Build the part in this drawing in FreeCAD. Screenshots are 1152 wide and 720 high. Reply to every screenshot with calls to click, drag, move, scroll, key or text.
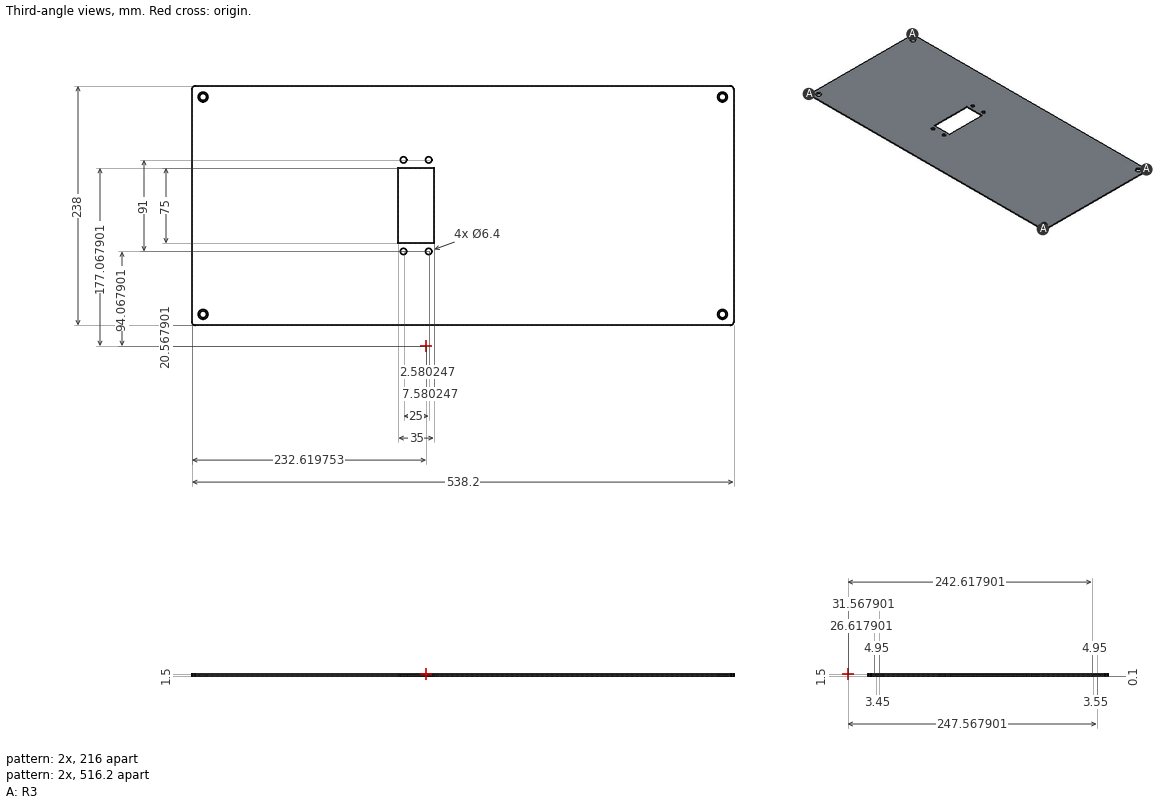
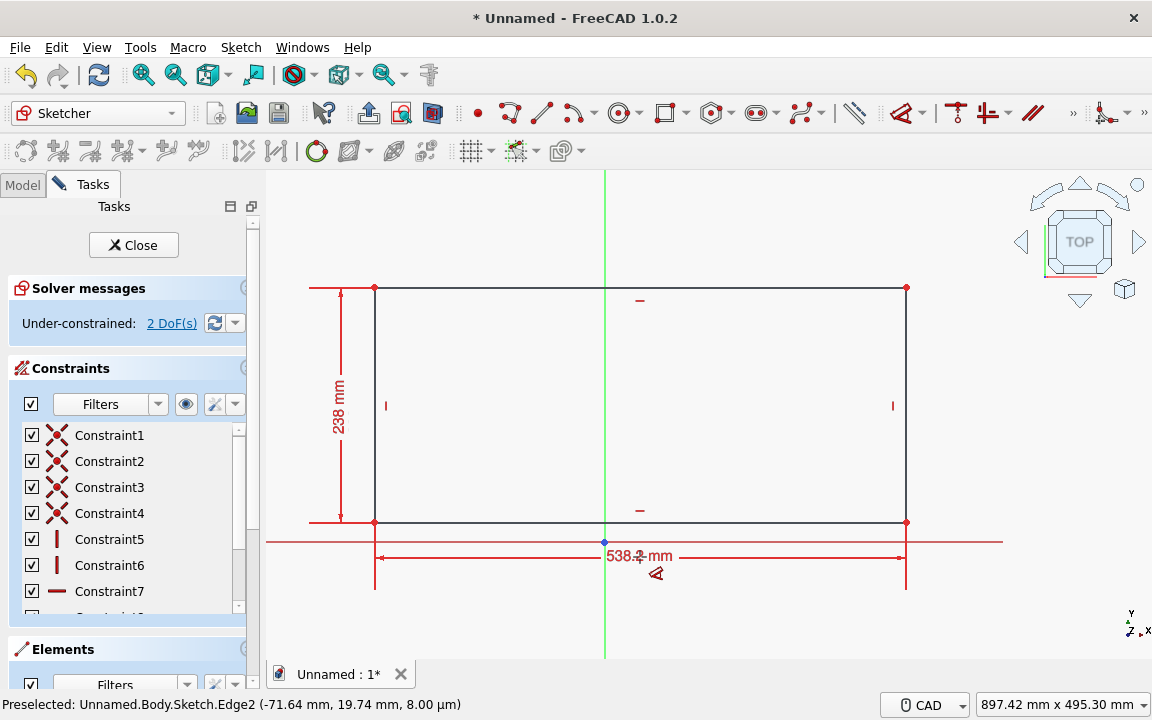
scroll(375, 523, up, 4)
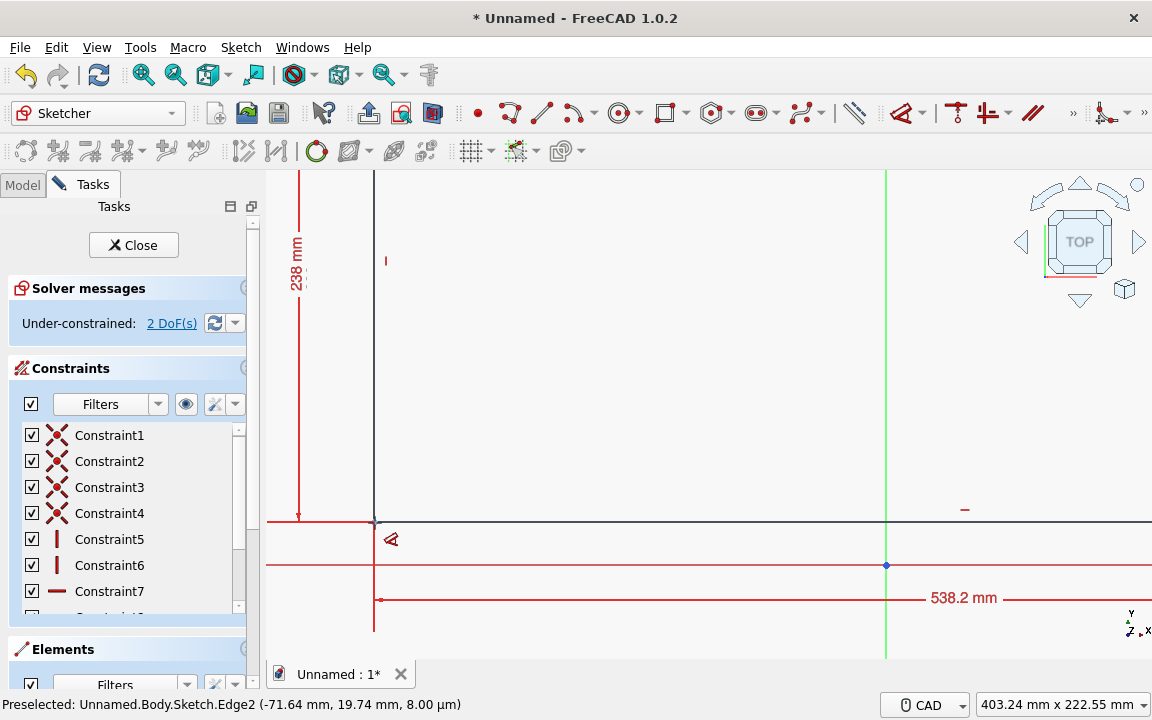
click(374, 522)
click(340, 544)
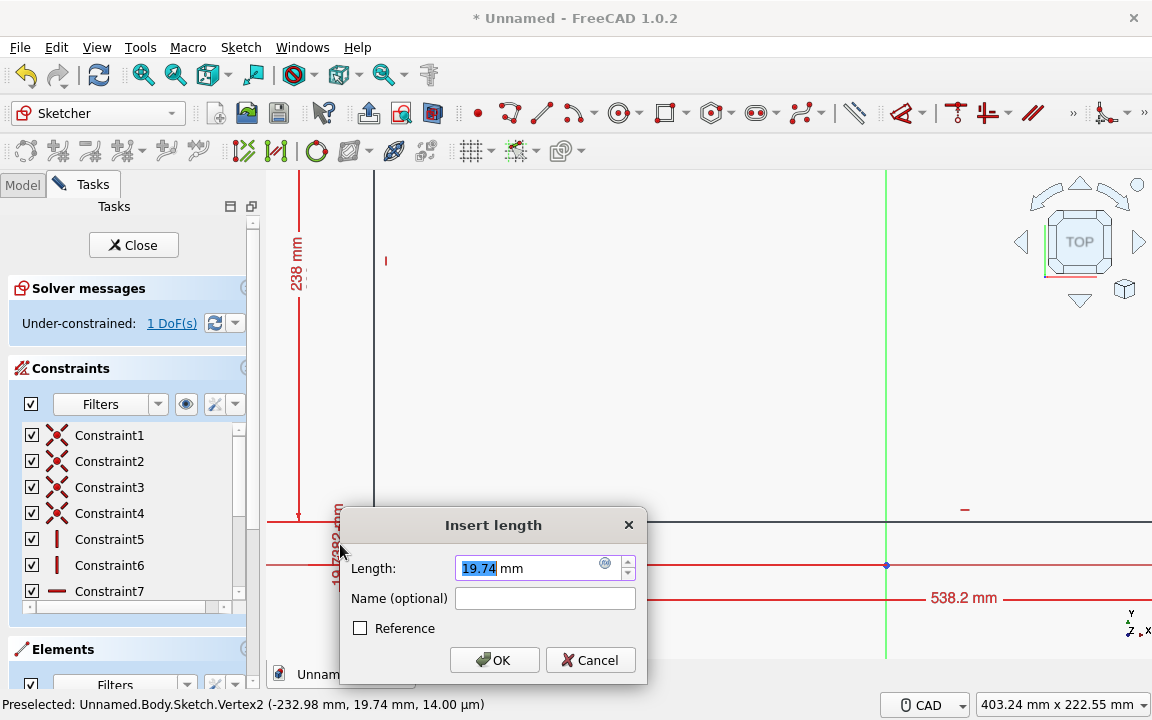
text(20.567901)
key(Return)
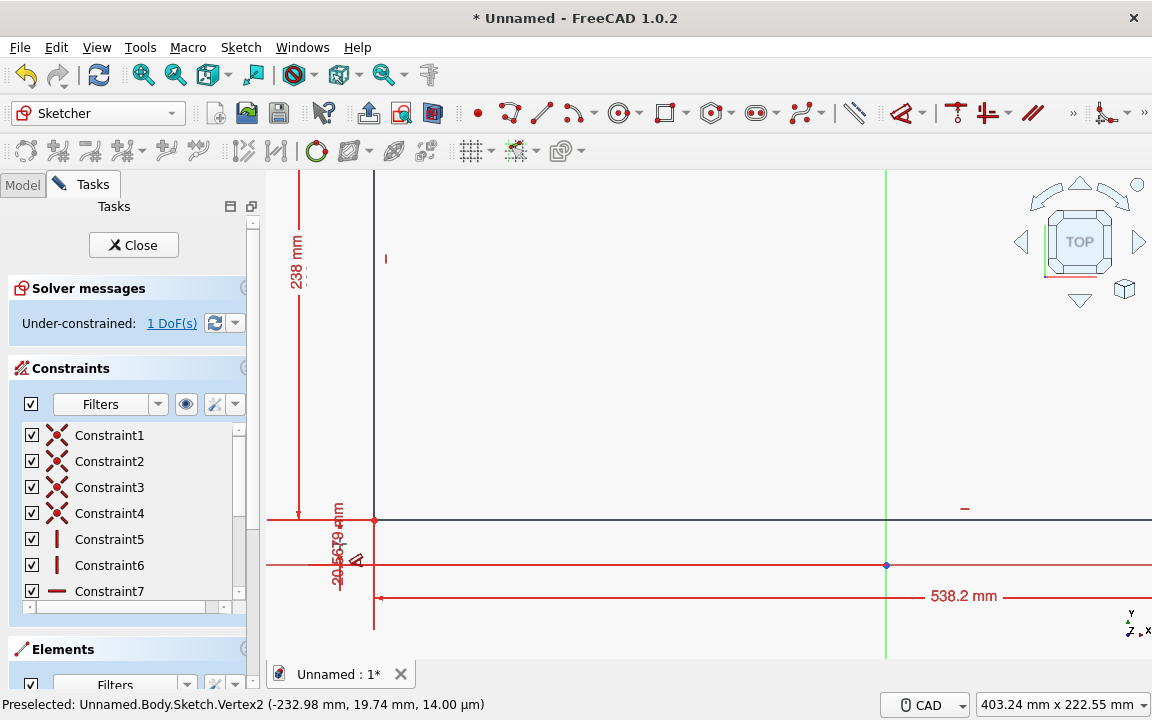
scroll(375, 523, down, 4)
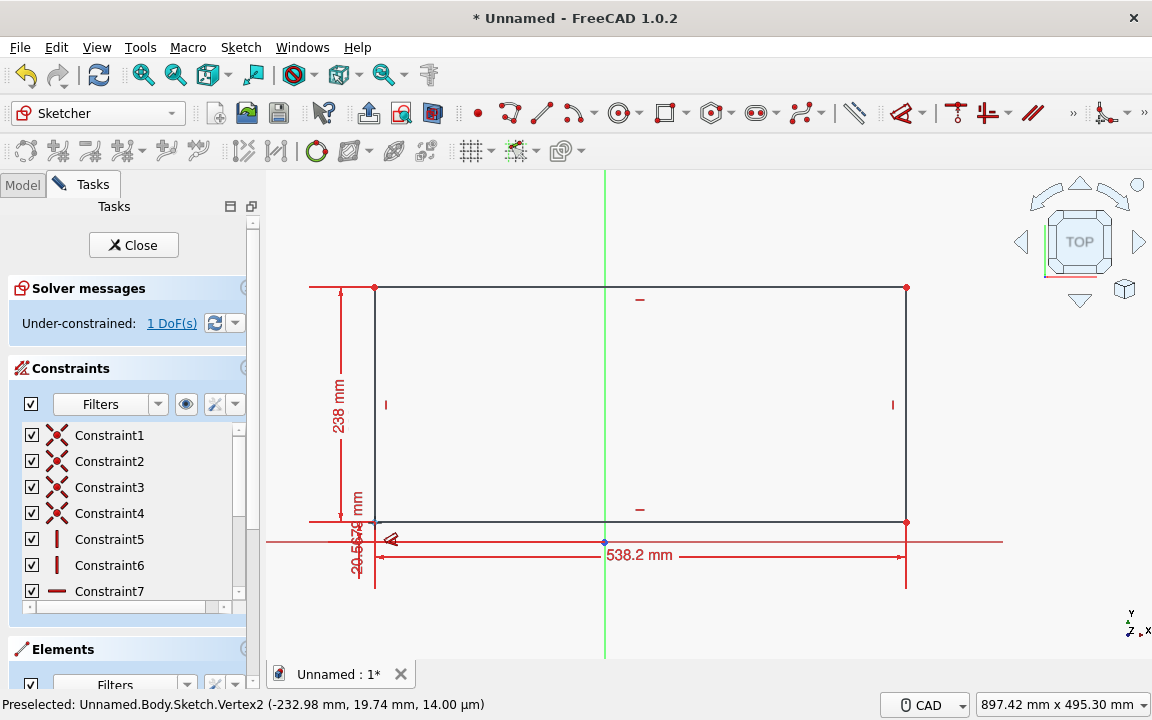
click(375, 287)
click(490, 576)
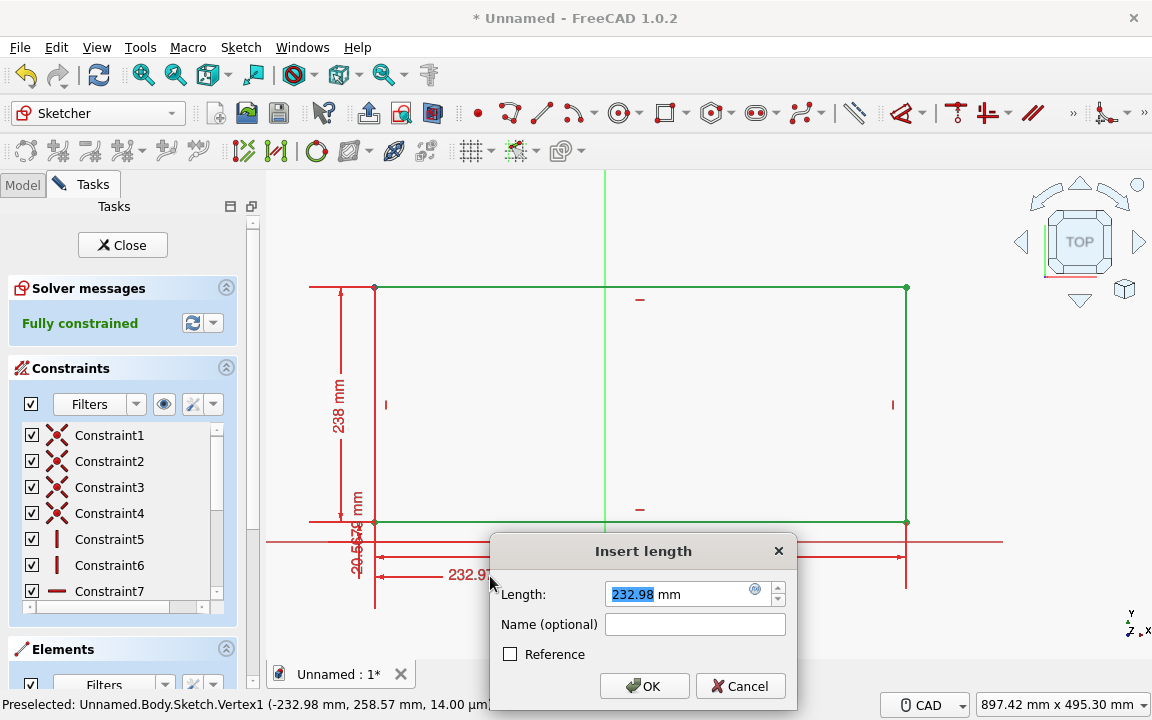
text(232.619753)
key(Return)
key(Escape)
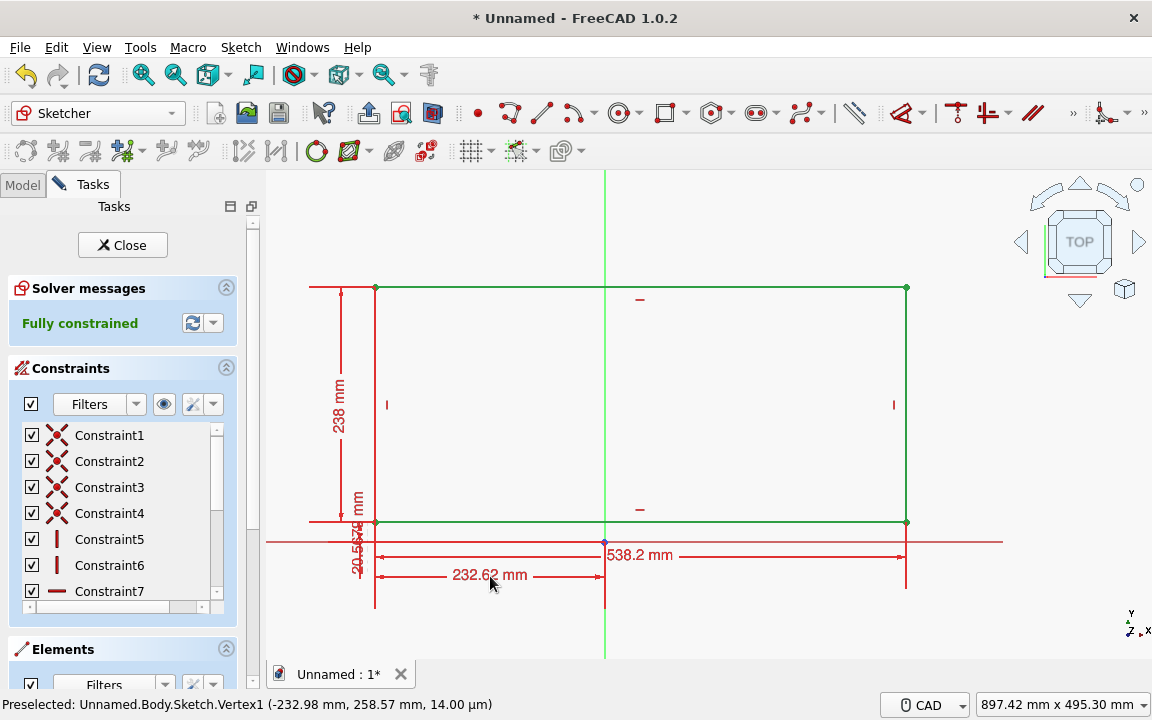
click(123, 245)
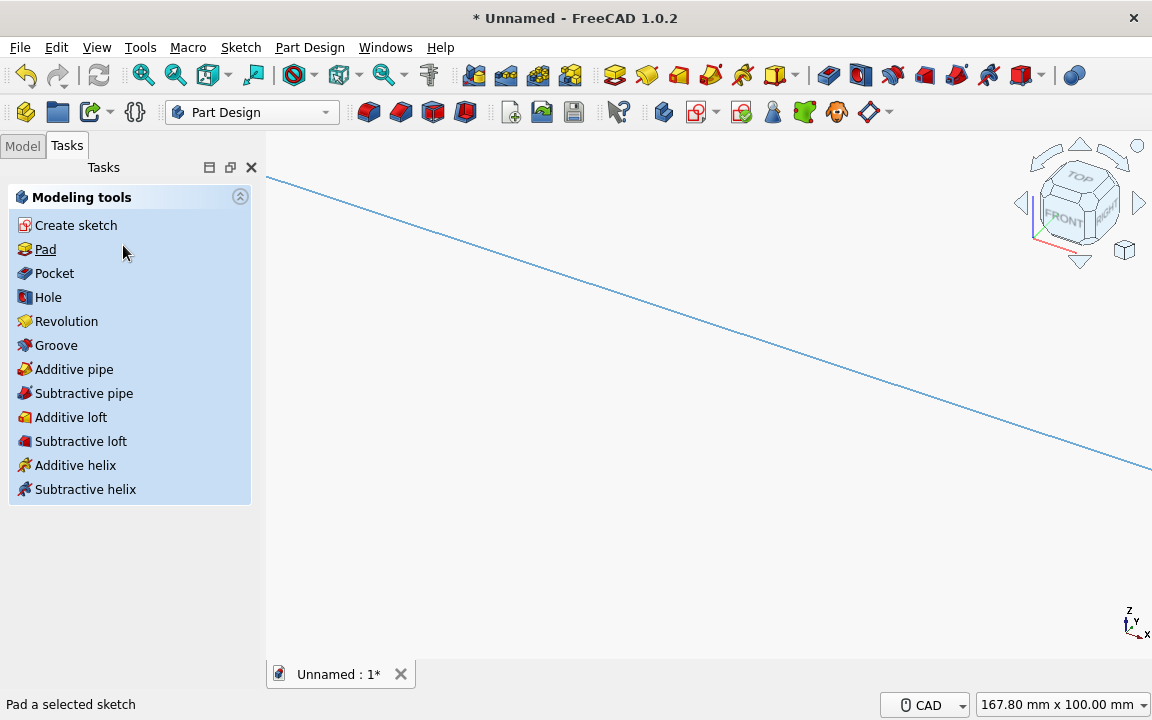
click(616, 76)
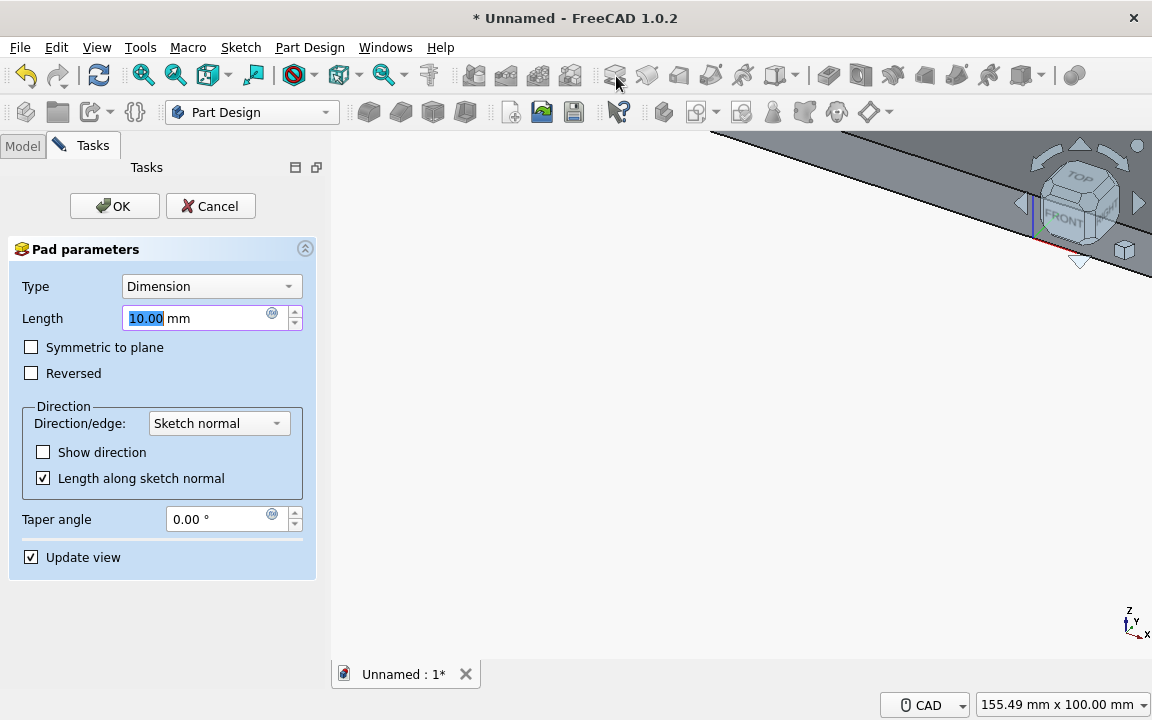
text(1.5)
key(Tab)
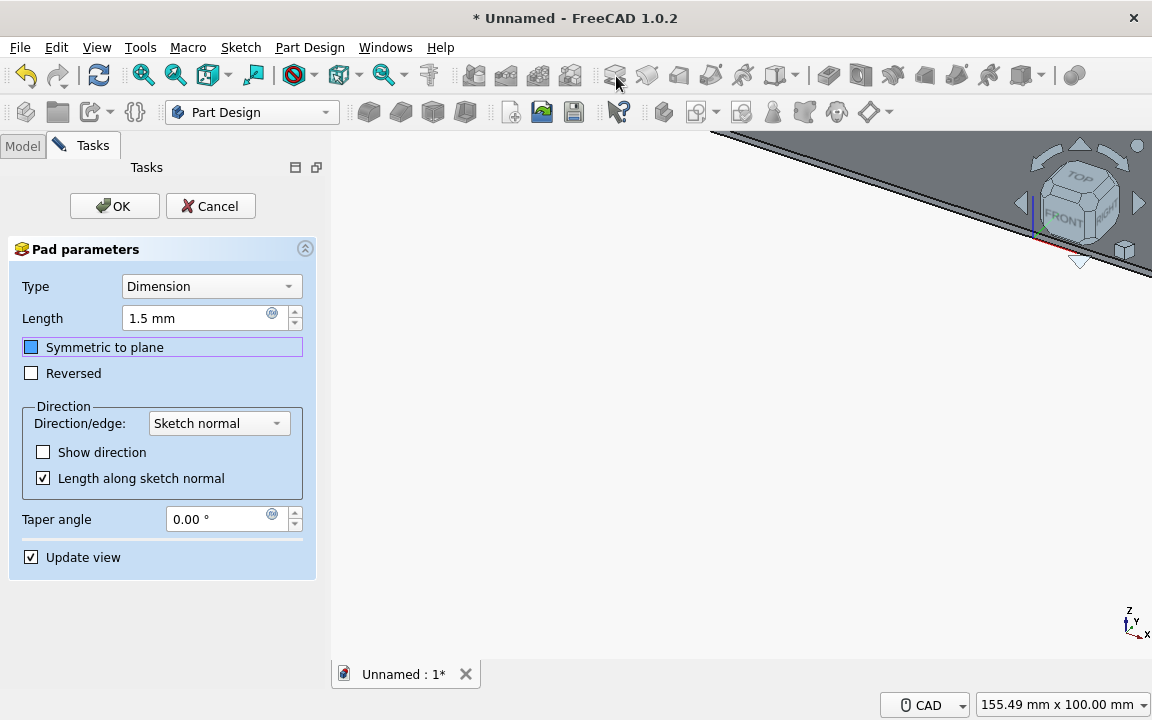
click(30, 373)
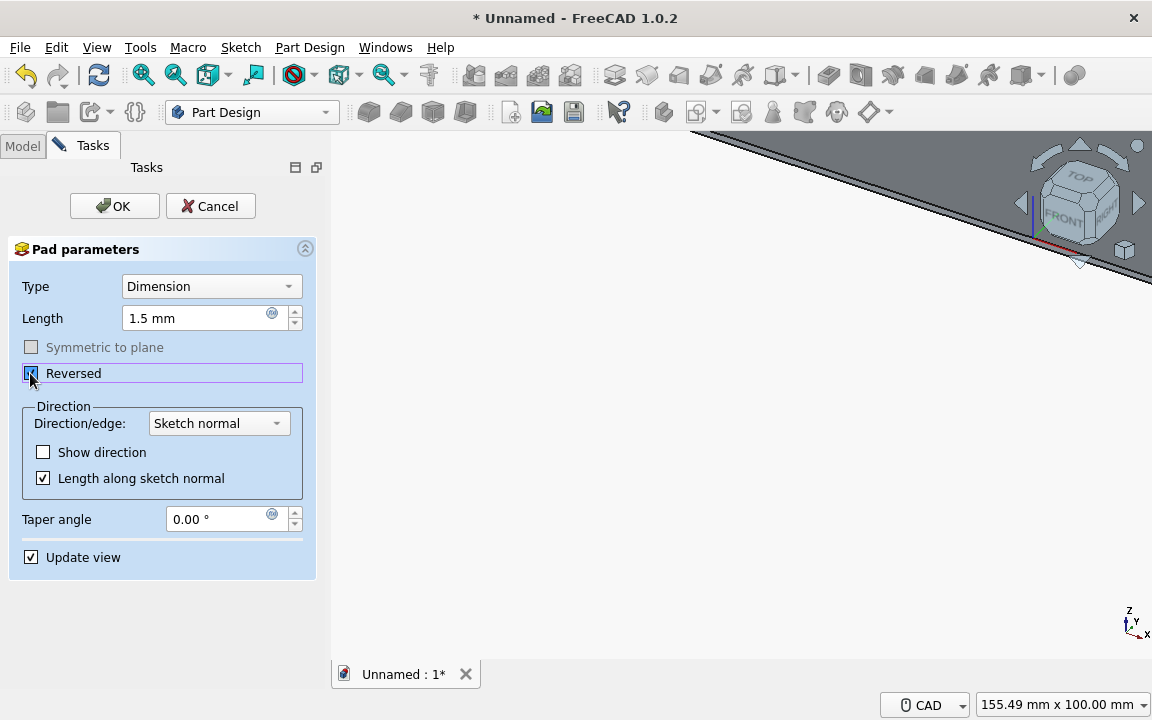
click(115, 206)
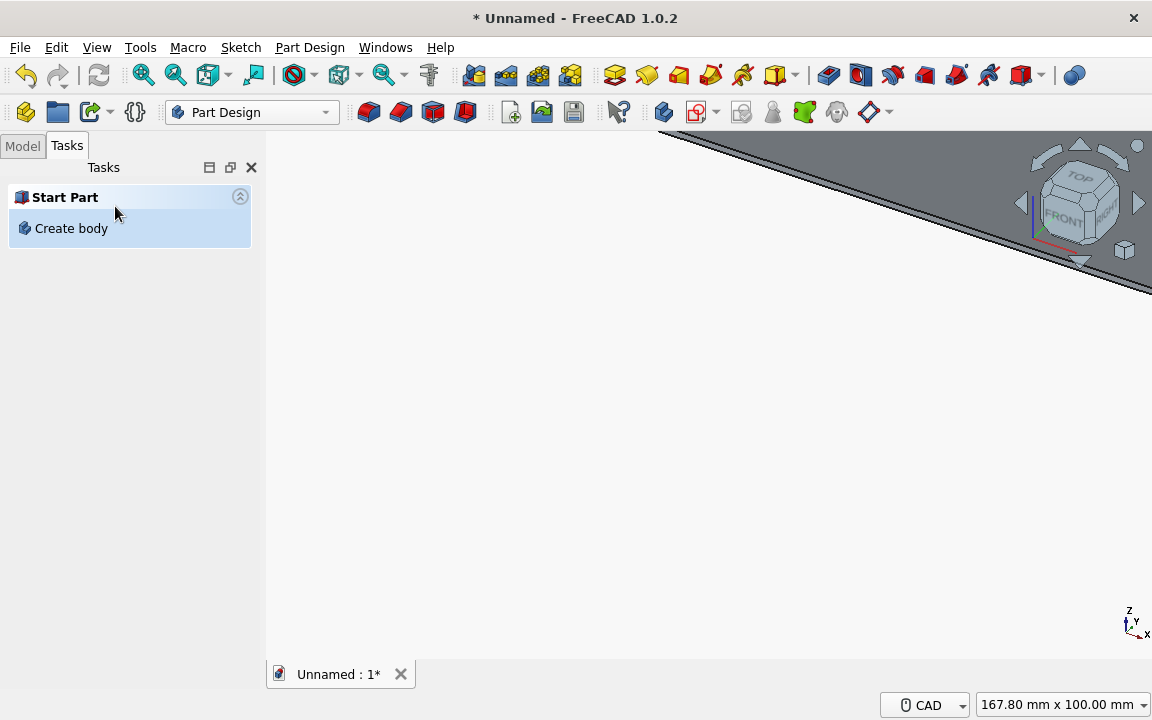
click(144, 76)